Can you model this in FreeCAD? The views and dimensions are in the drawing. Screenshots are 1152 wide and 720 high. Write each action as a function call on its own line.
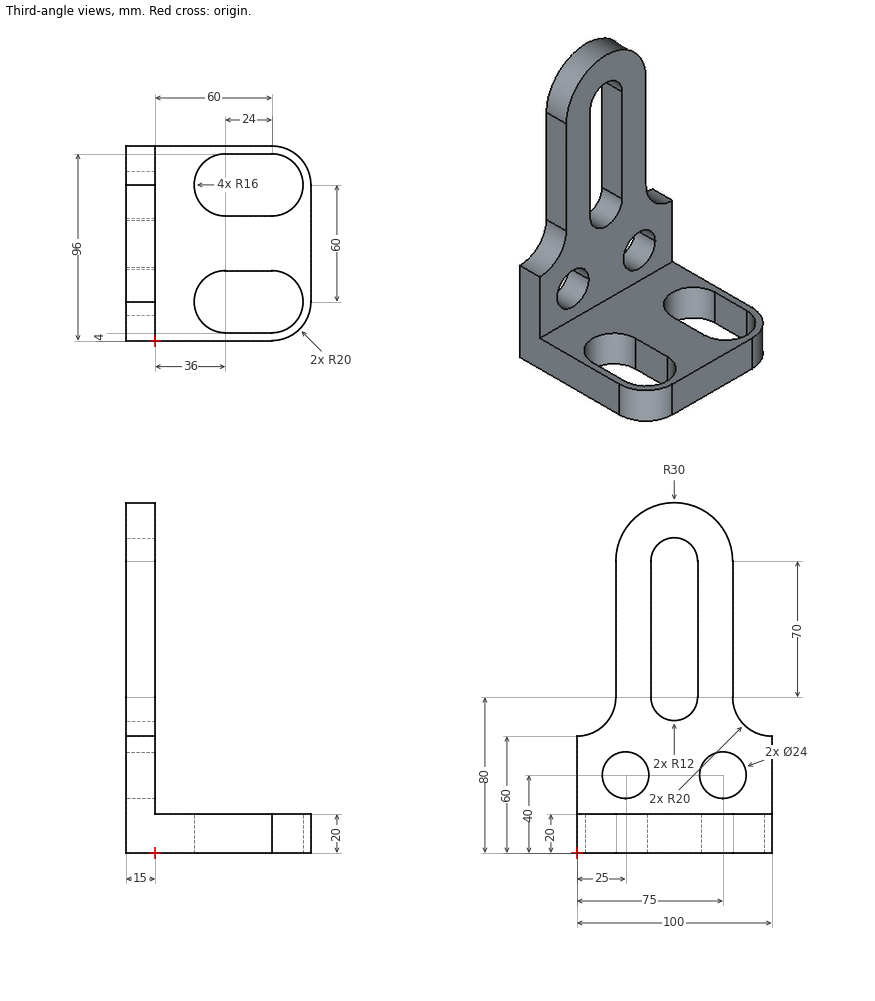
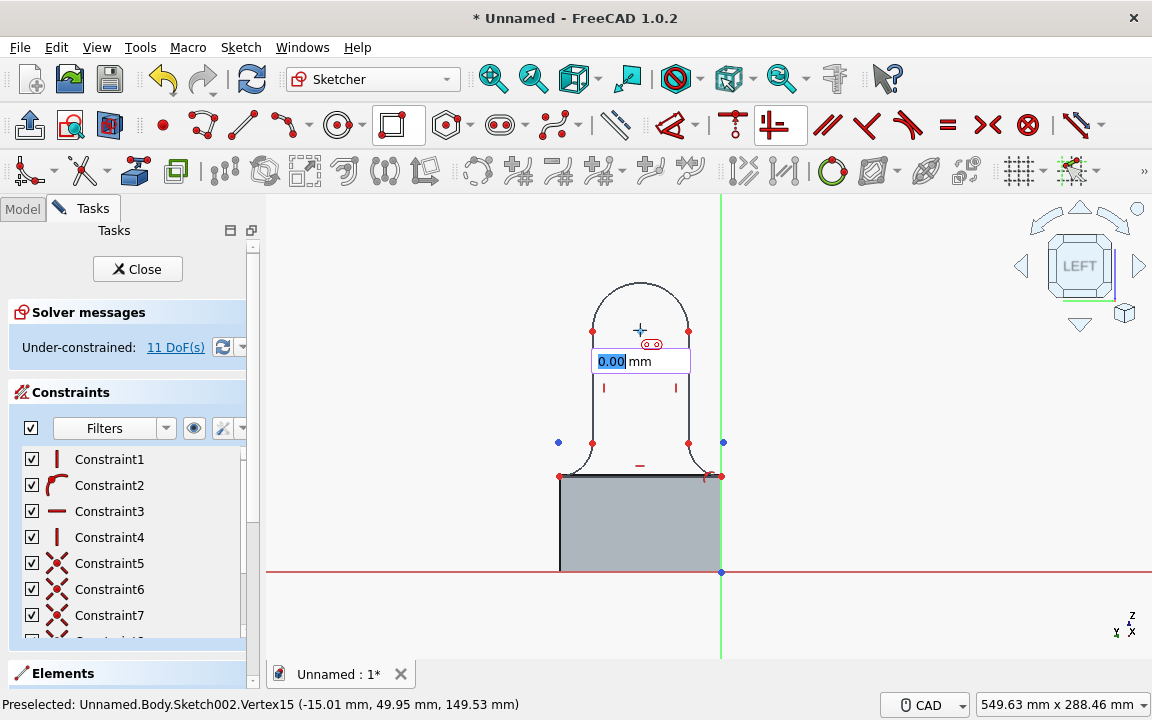
click(621, 387)
key(Escape)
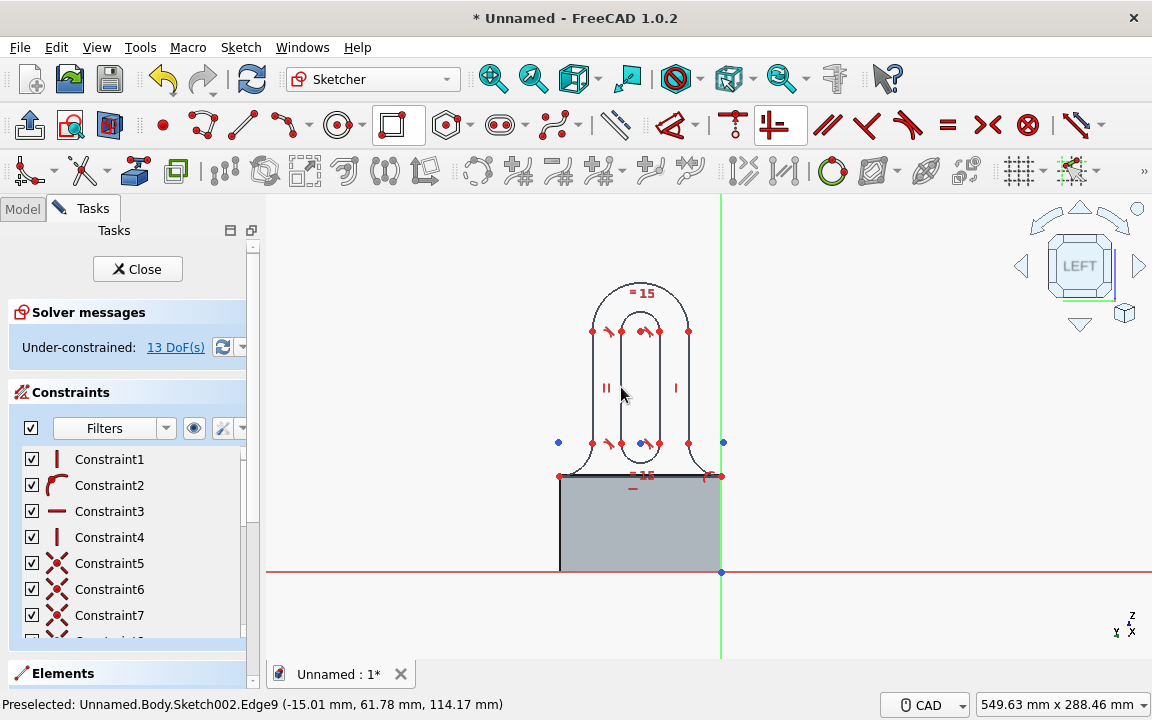
click(593, 365)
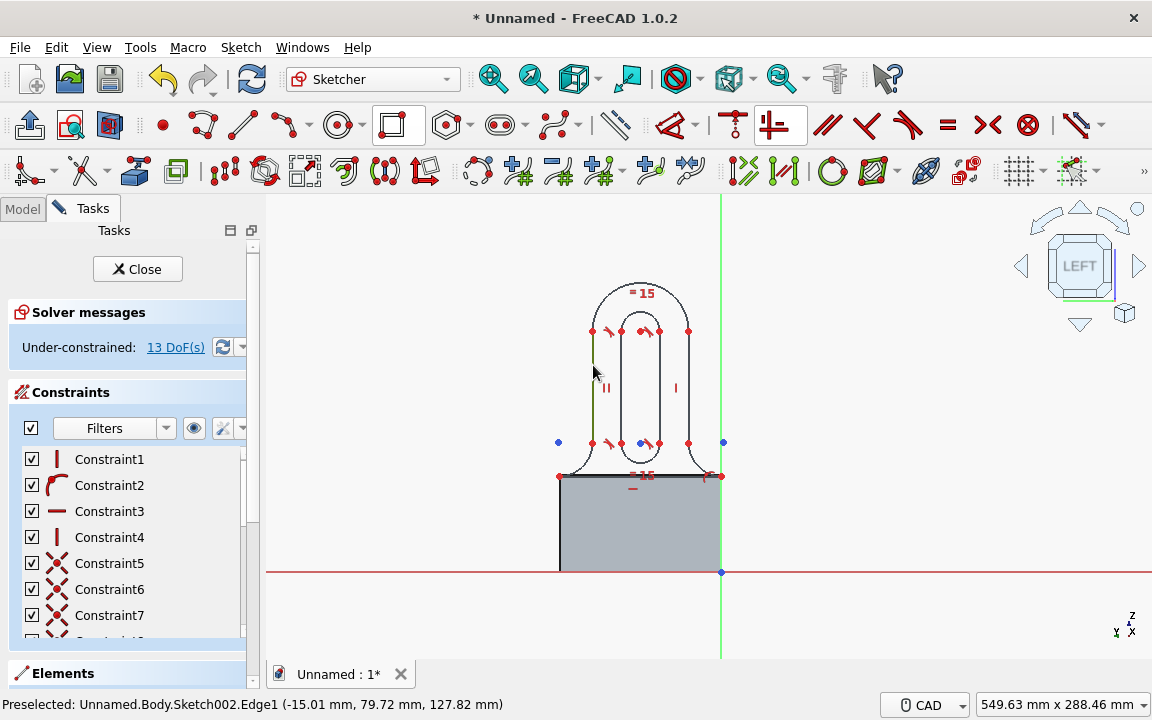
click(589, 458)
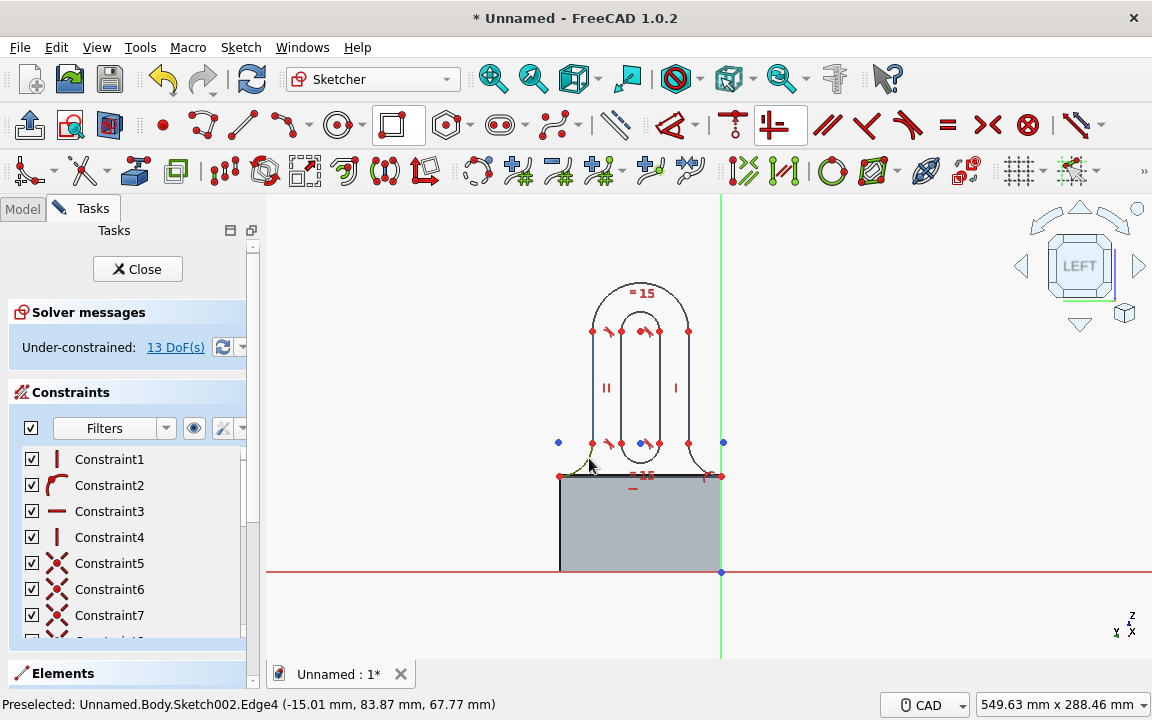
click(908, 126)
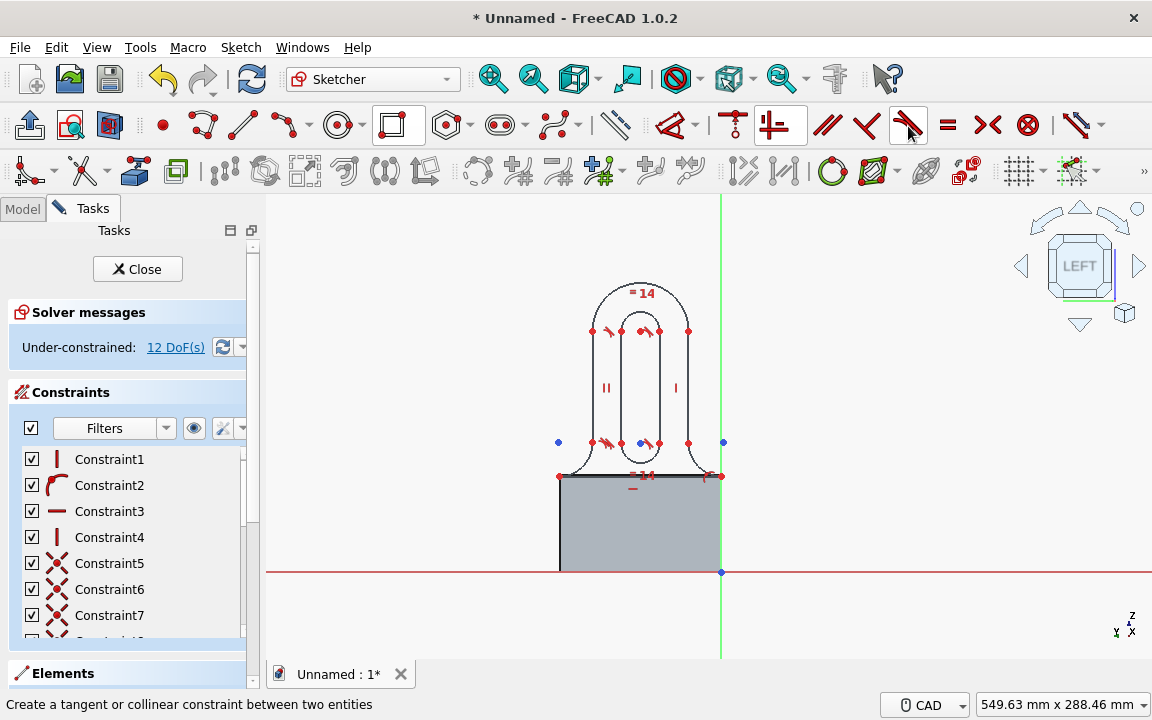
click(593, 365)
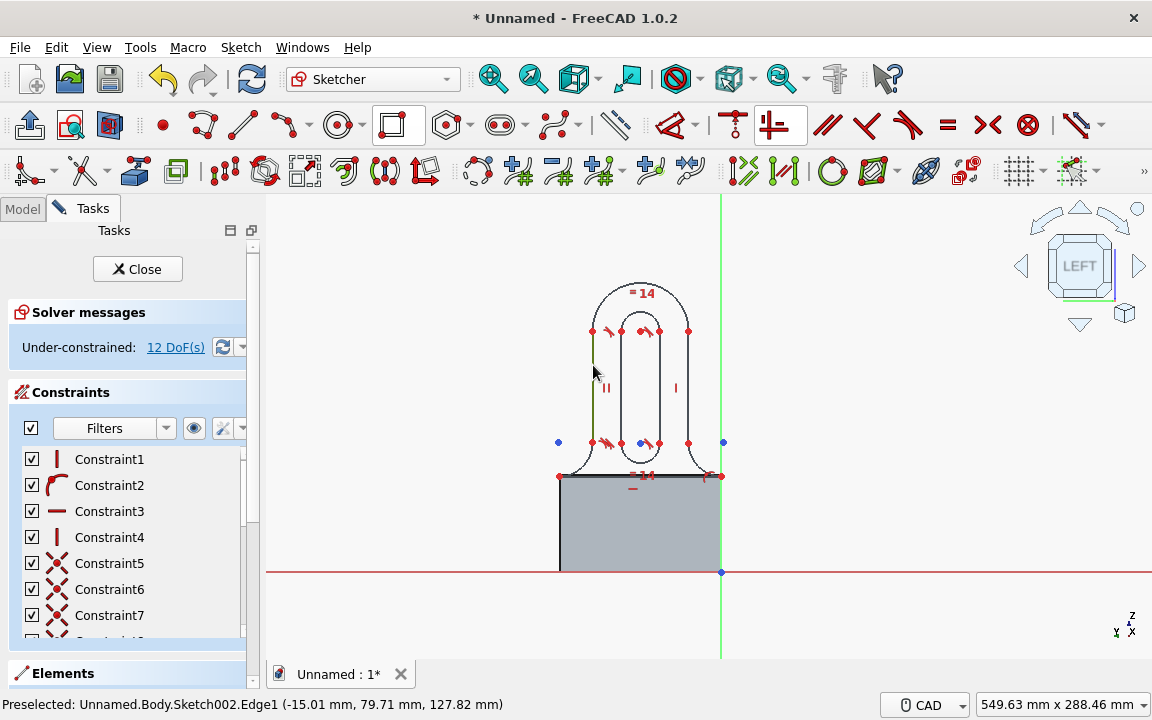
click(669, 292)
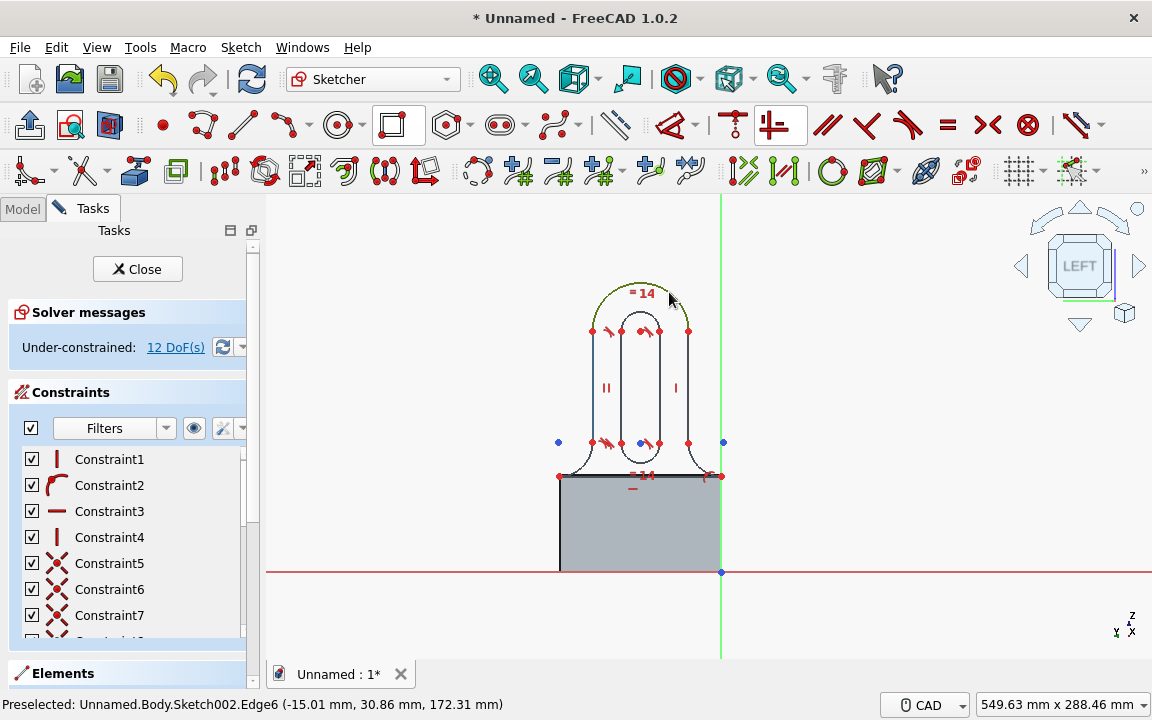
key(t)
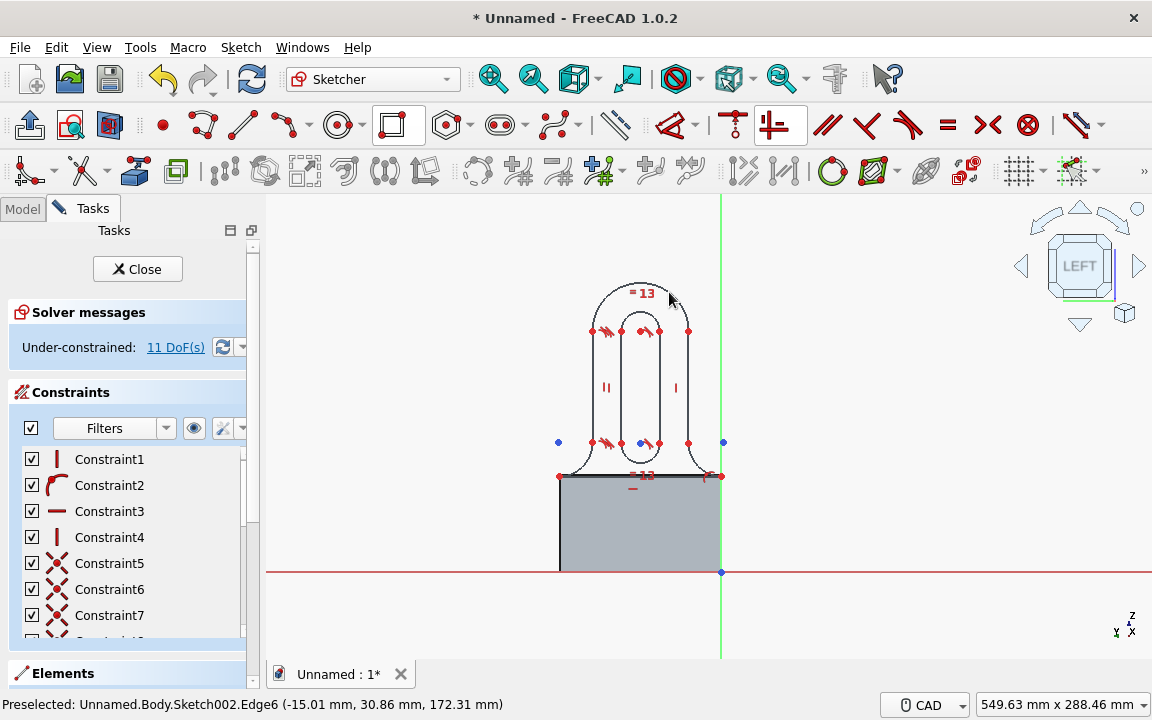
click(608, 477)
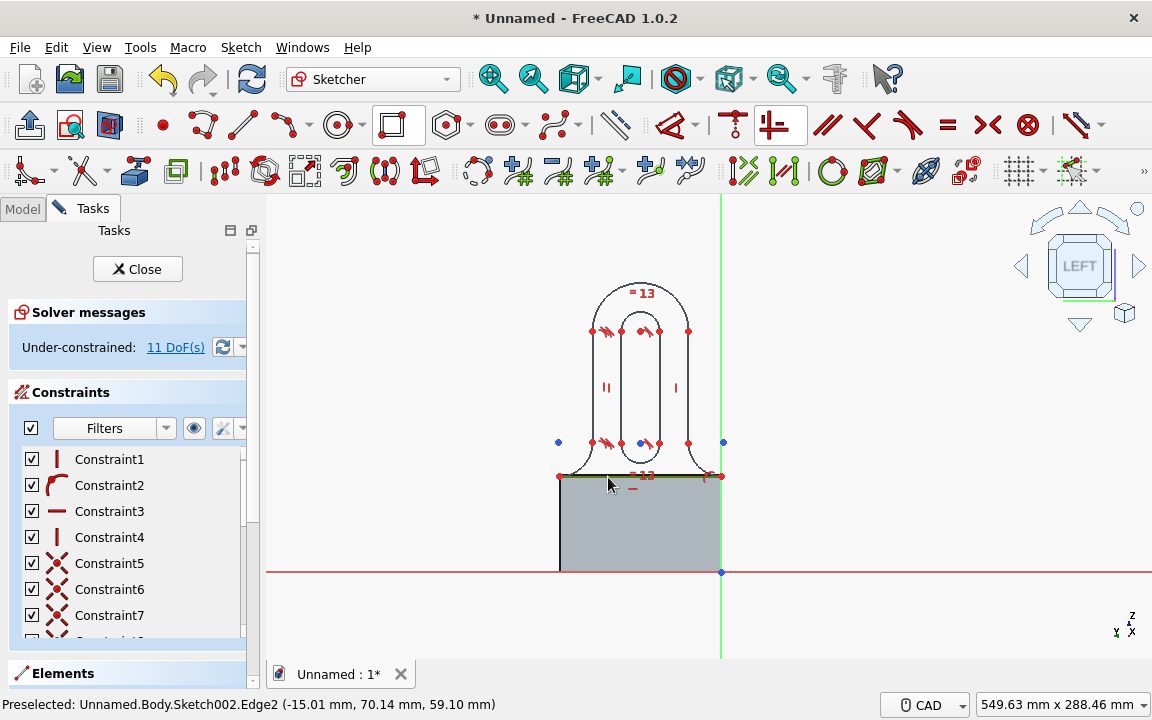
click(589, 458)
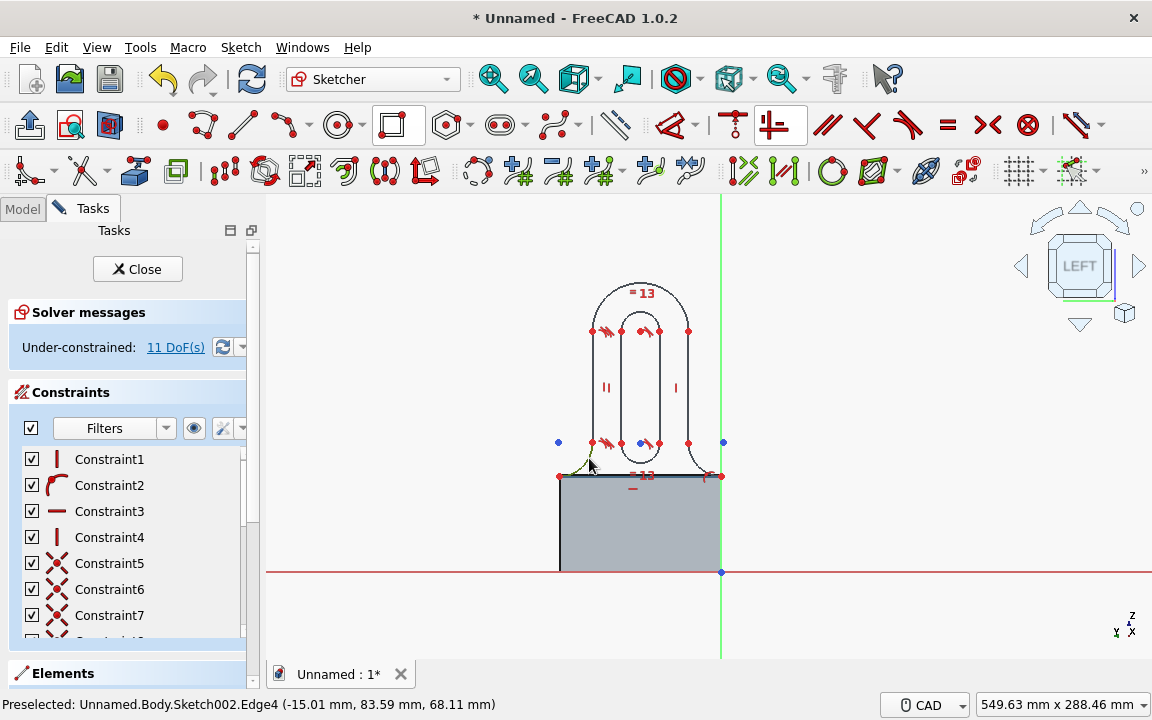
click(908, 126)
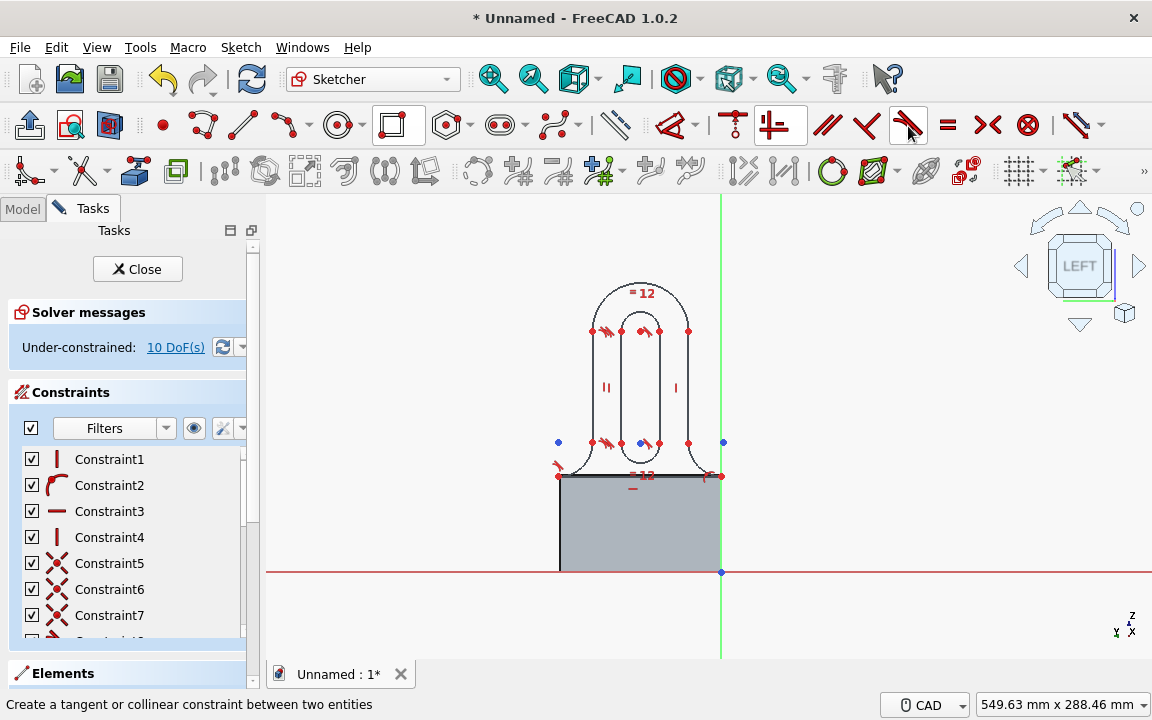
click(607, 477)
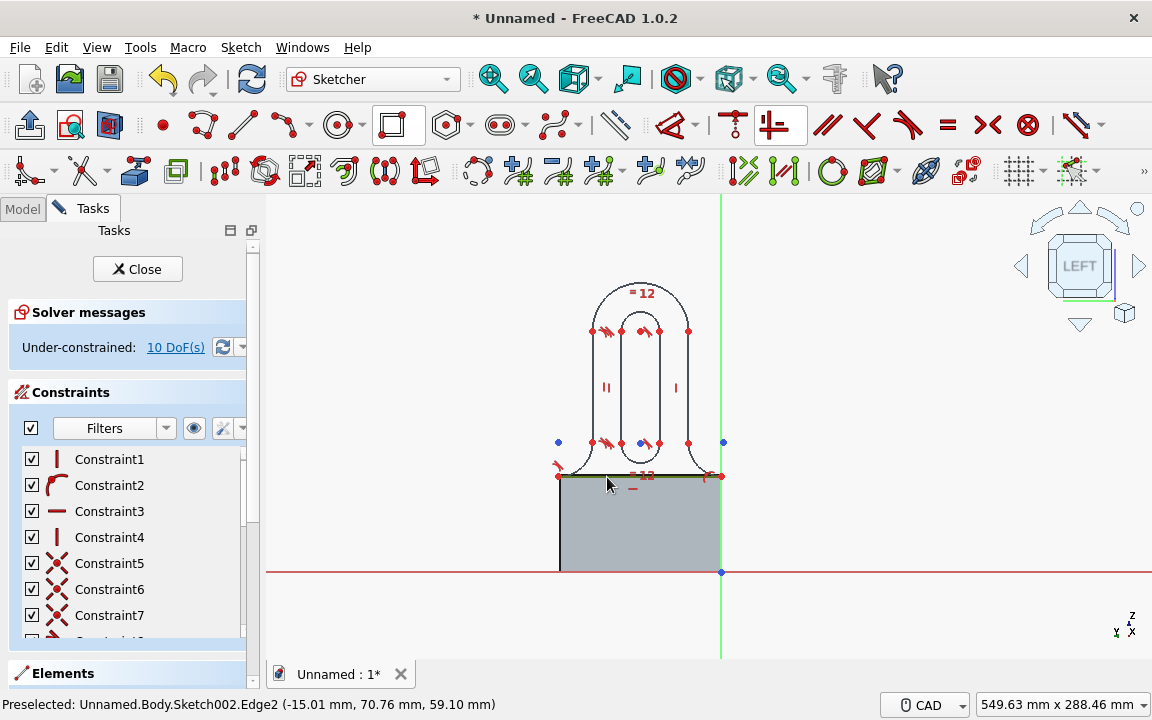
click(692, 458)